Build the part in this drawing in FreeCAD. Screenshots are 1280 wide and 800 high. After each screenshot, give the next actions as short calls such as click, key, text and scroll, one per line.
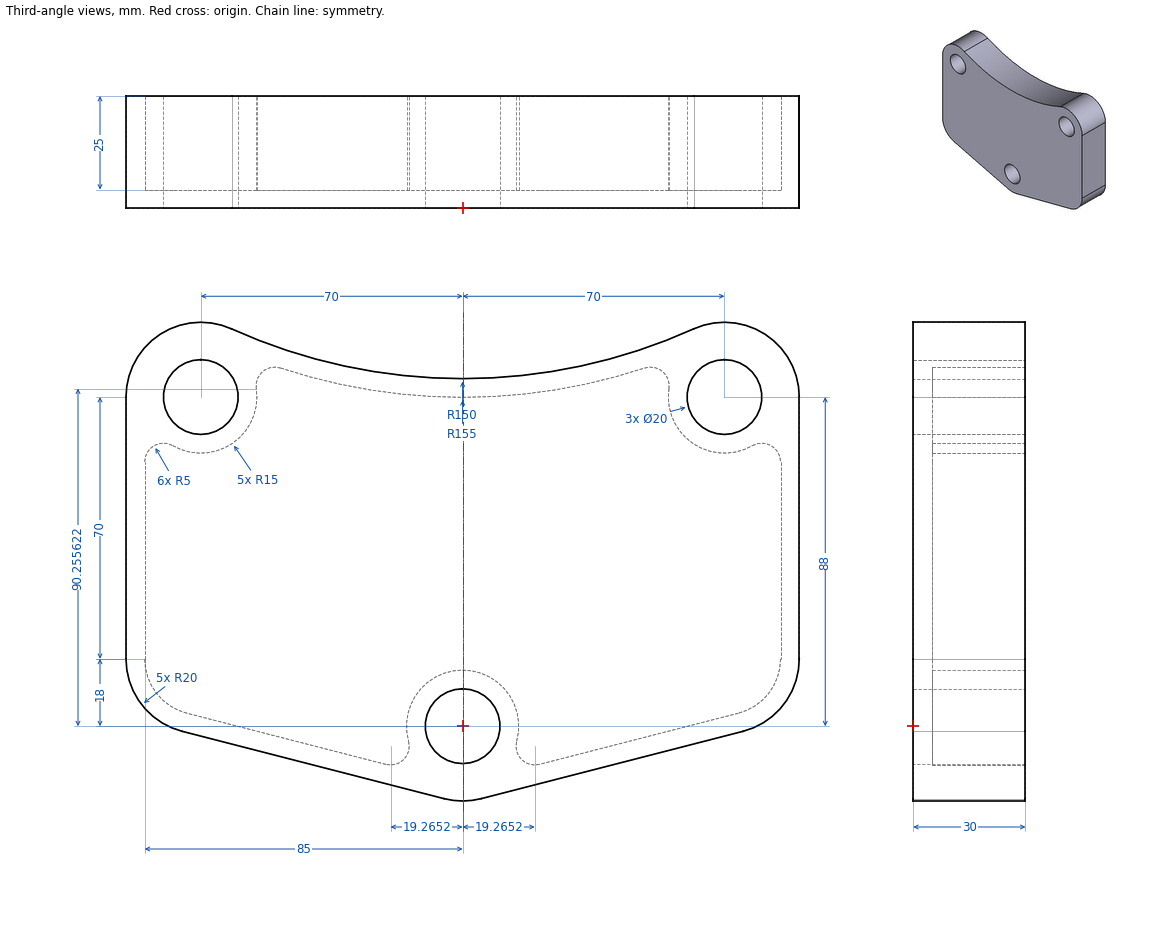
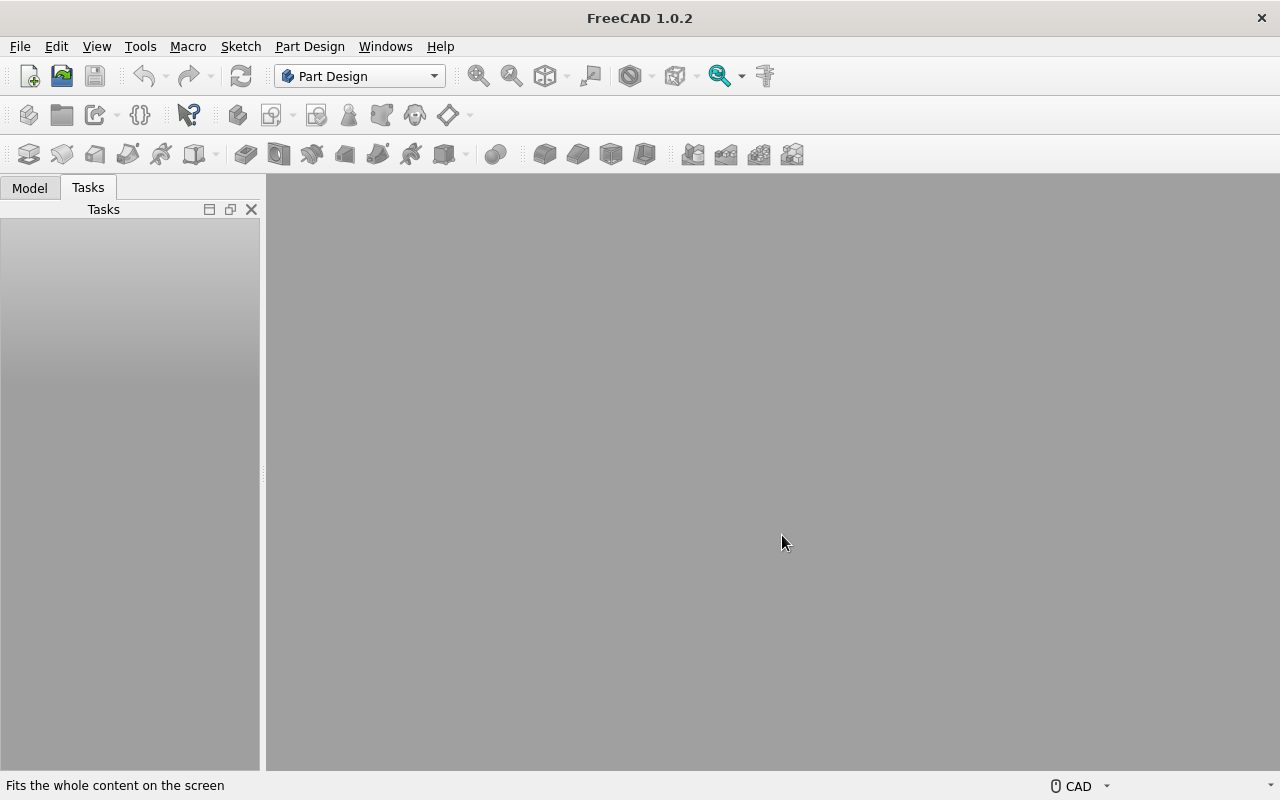
click(29, 76)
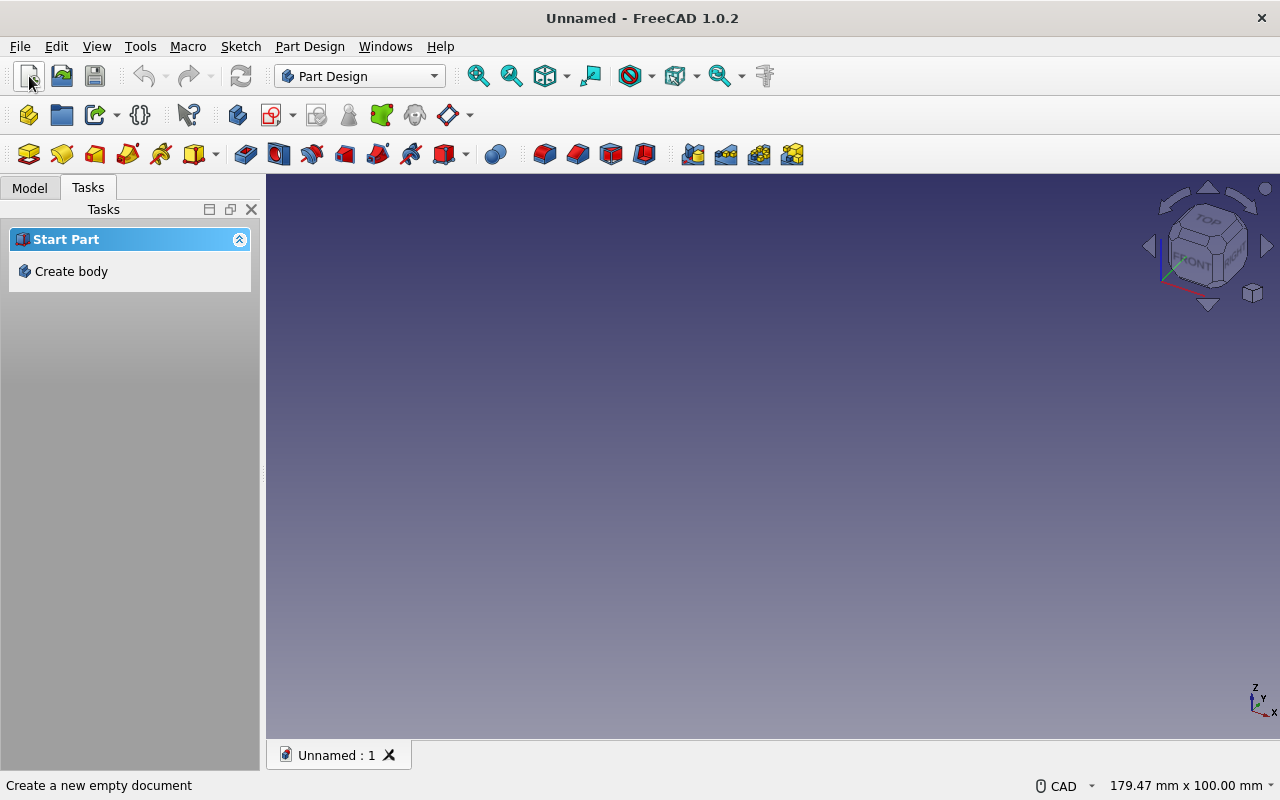
click(270, 116)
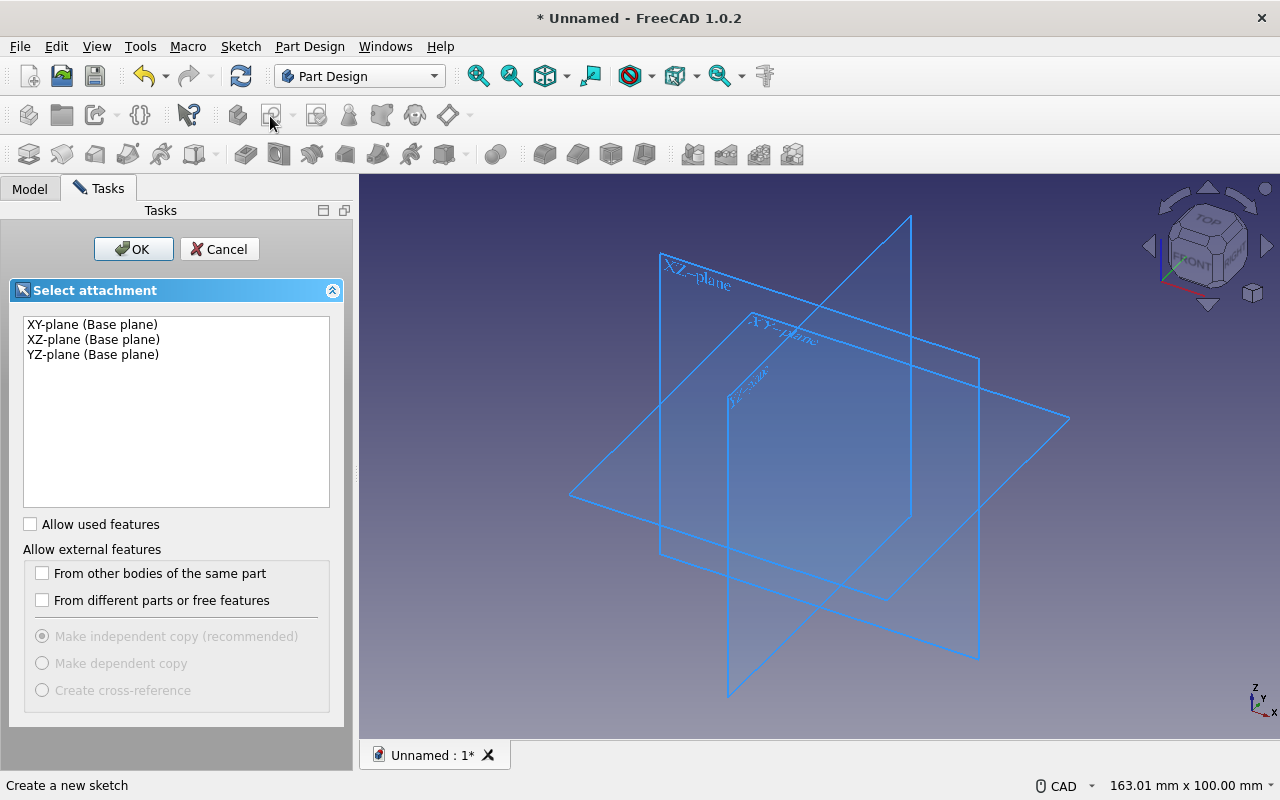
click(84, 340)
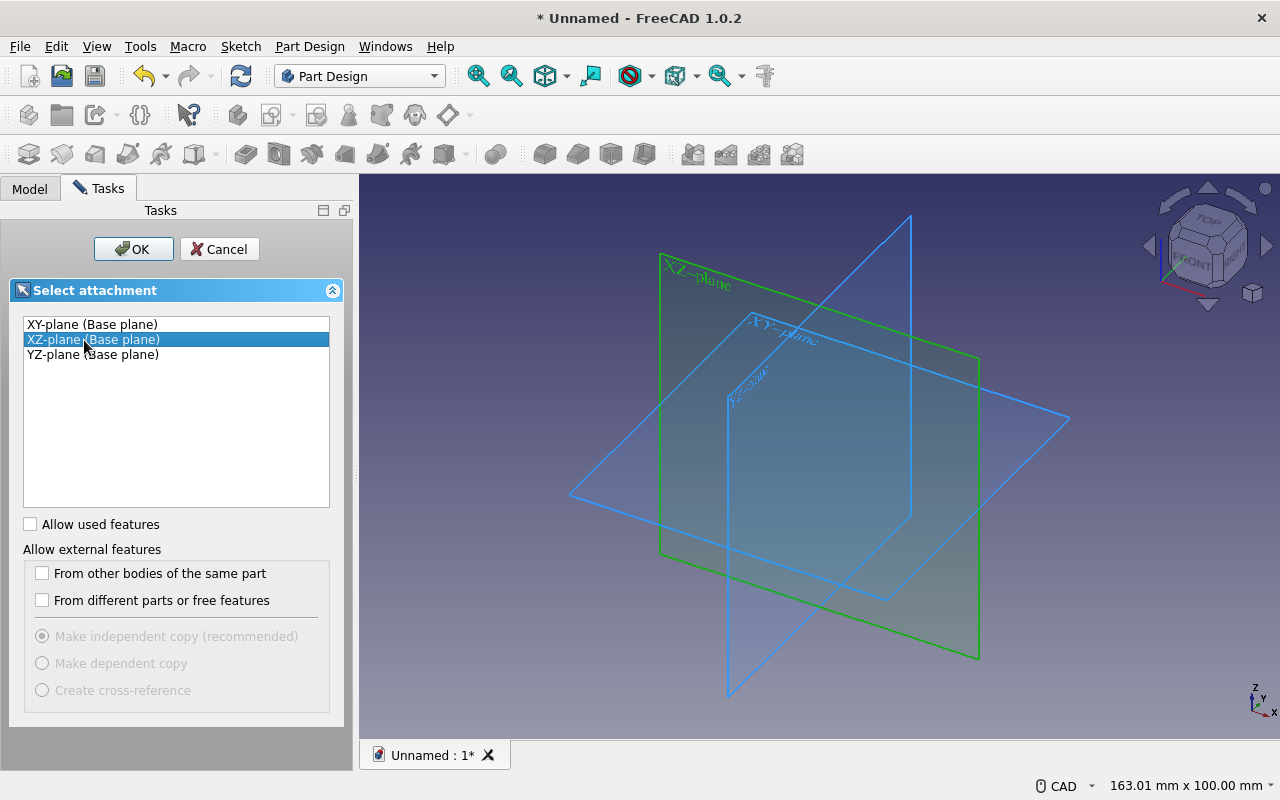
click(134, 249)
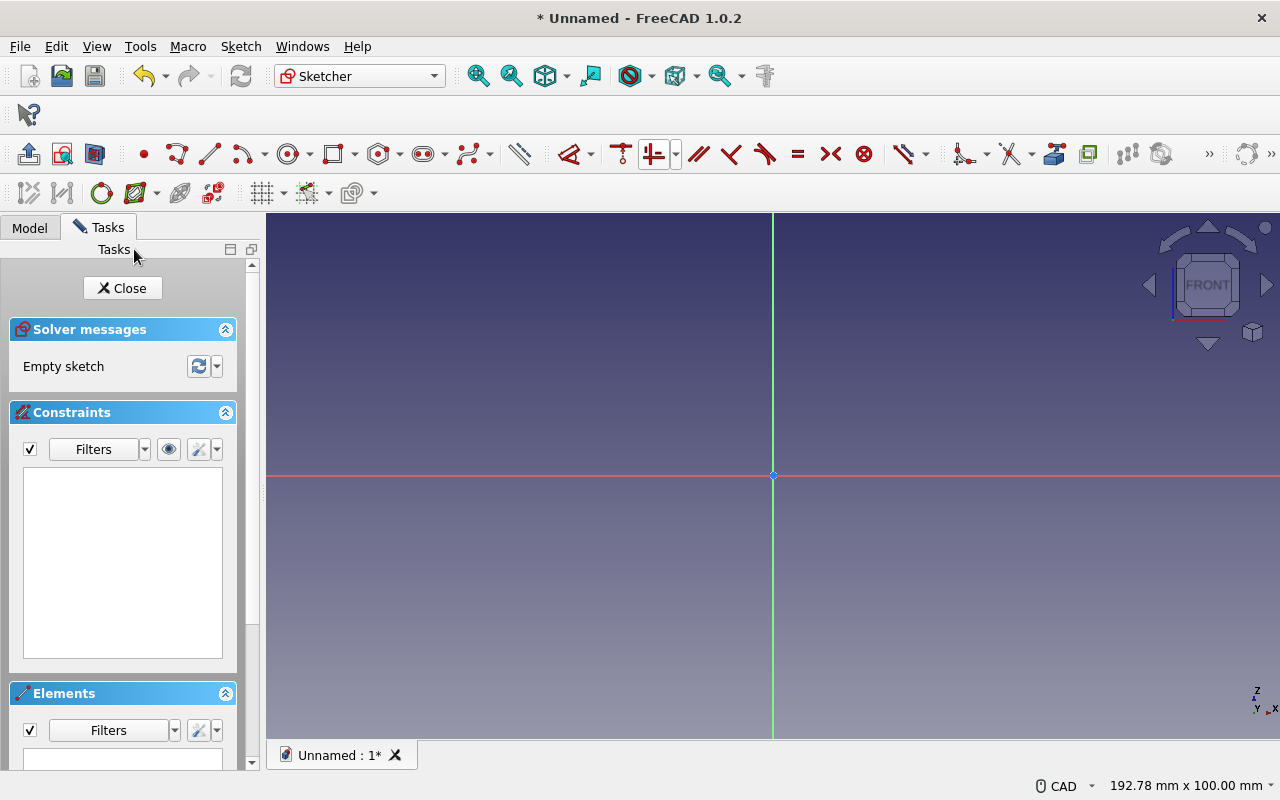
scroll(621, 711, down, 3)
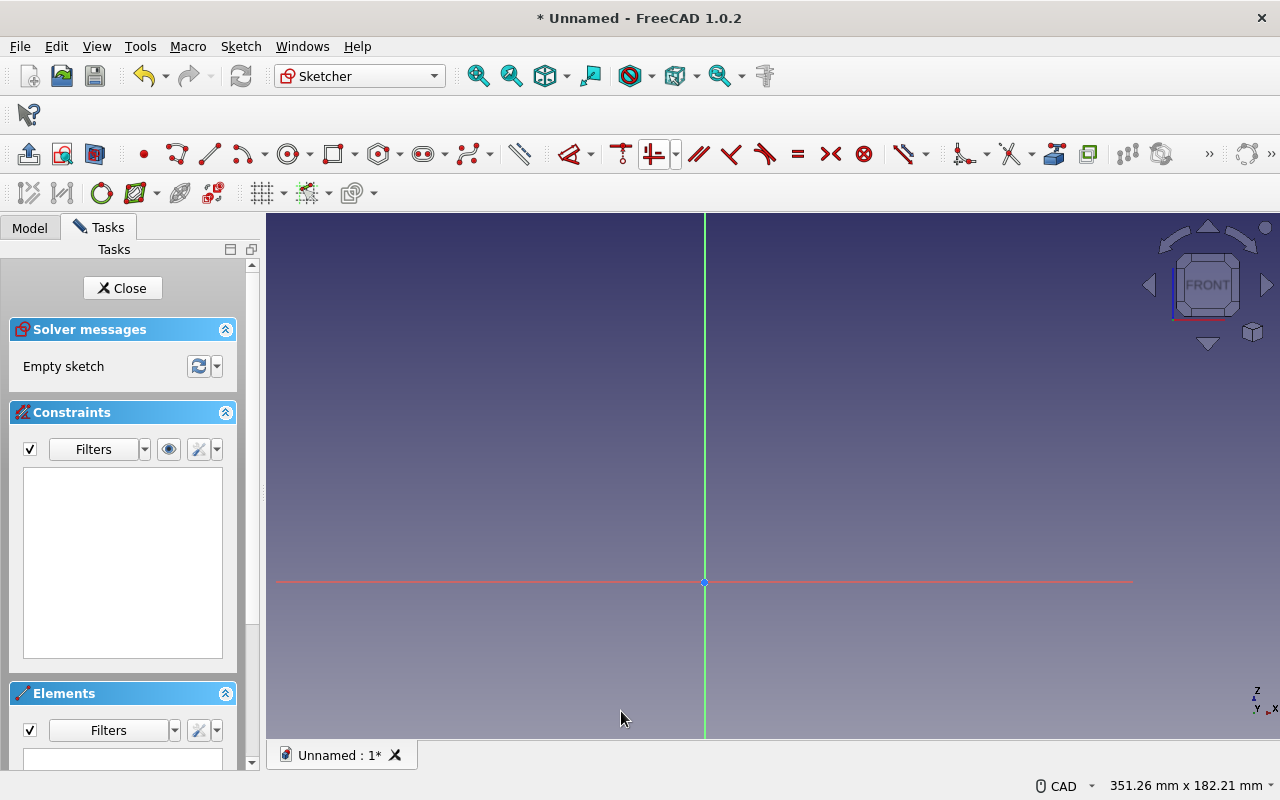
click(210, 154)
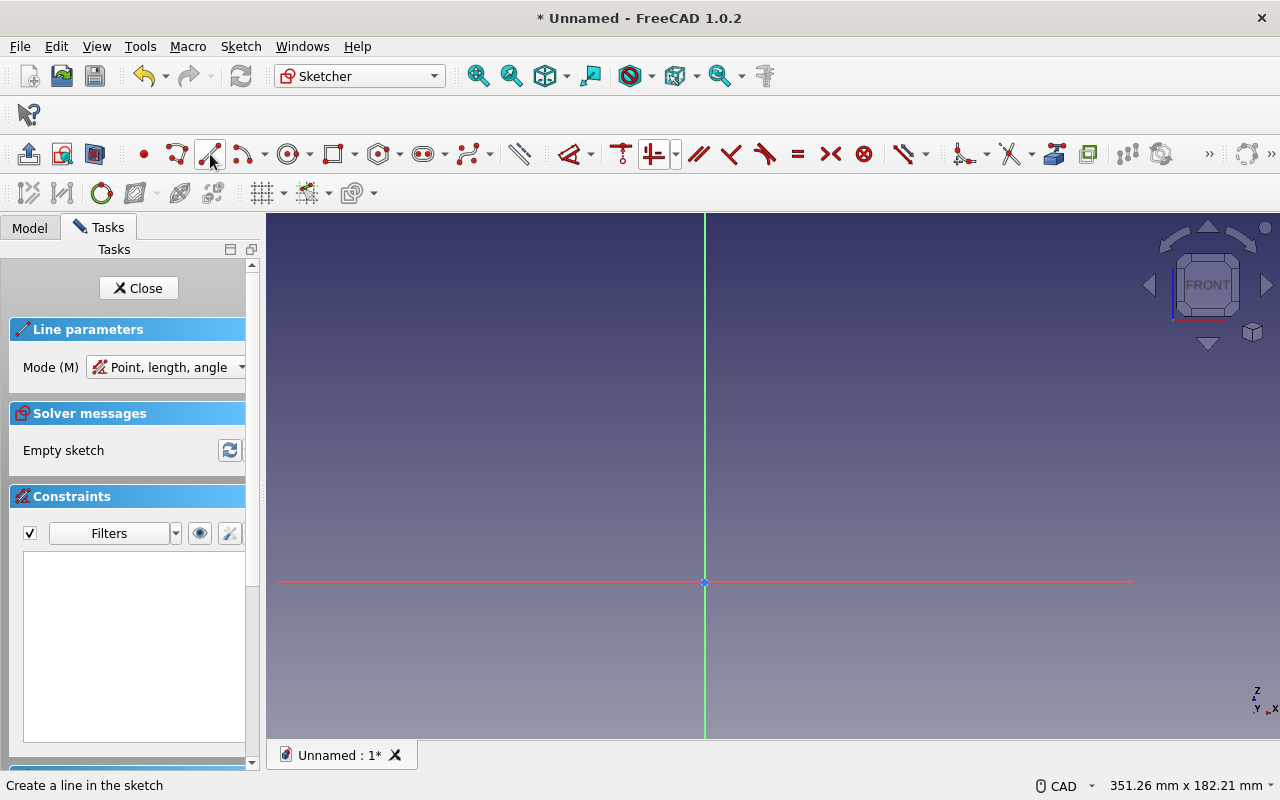
click(690, 638)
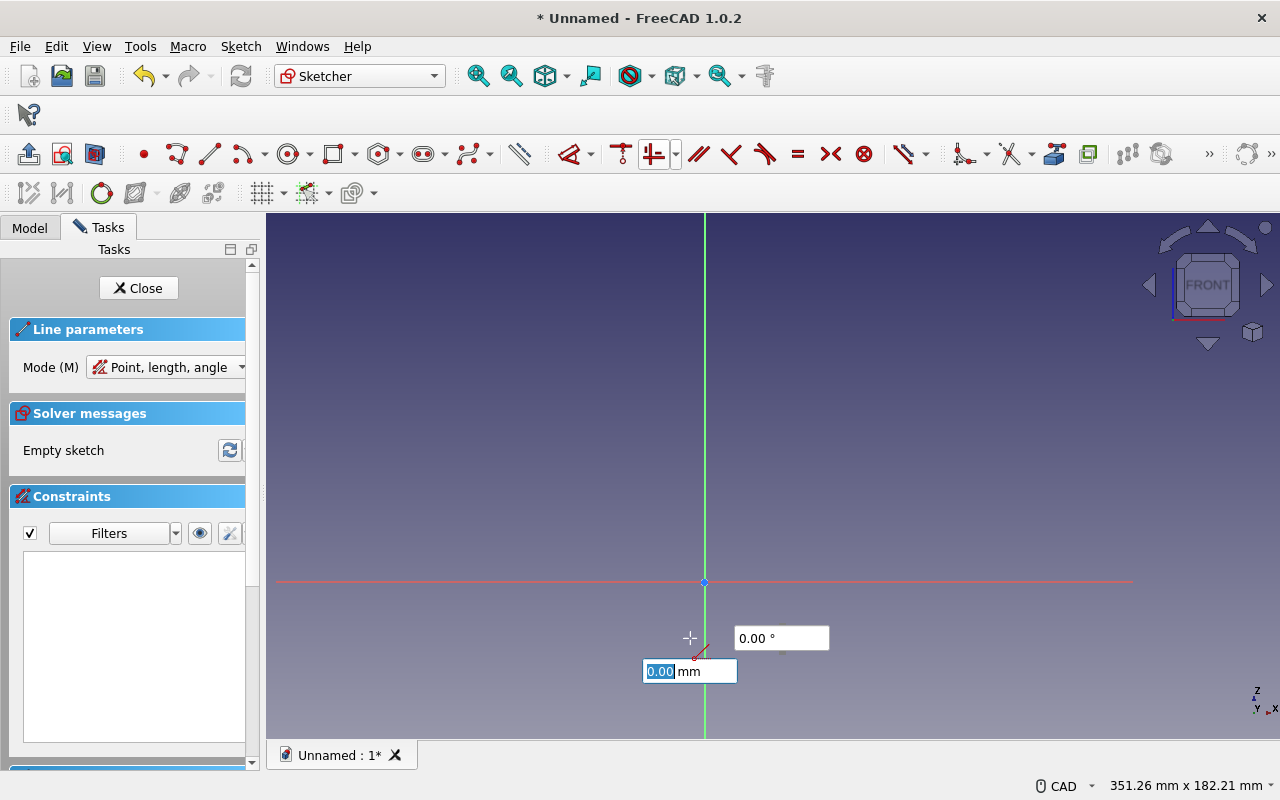
scroll(488, 586, up, 7)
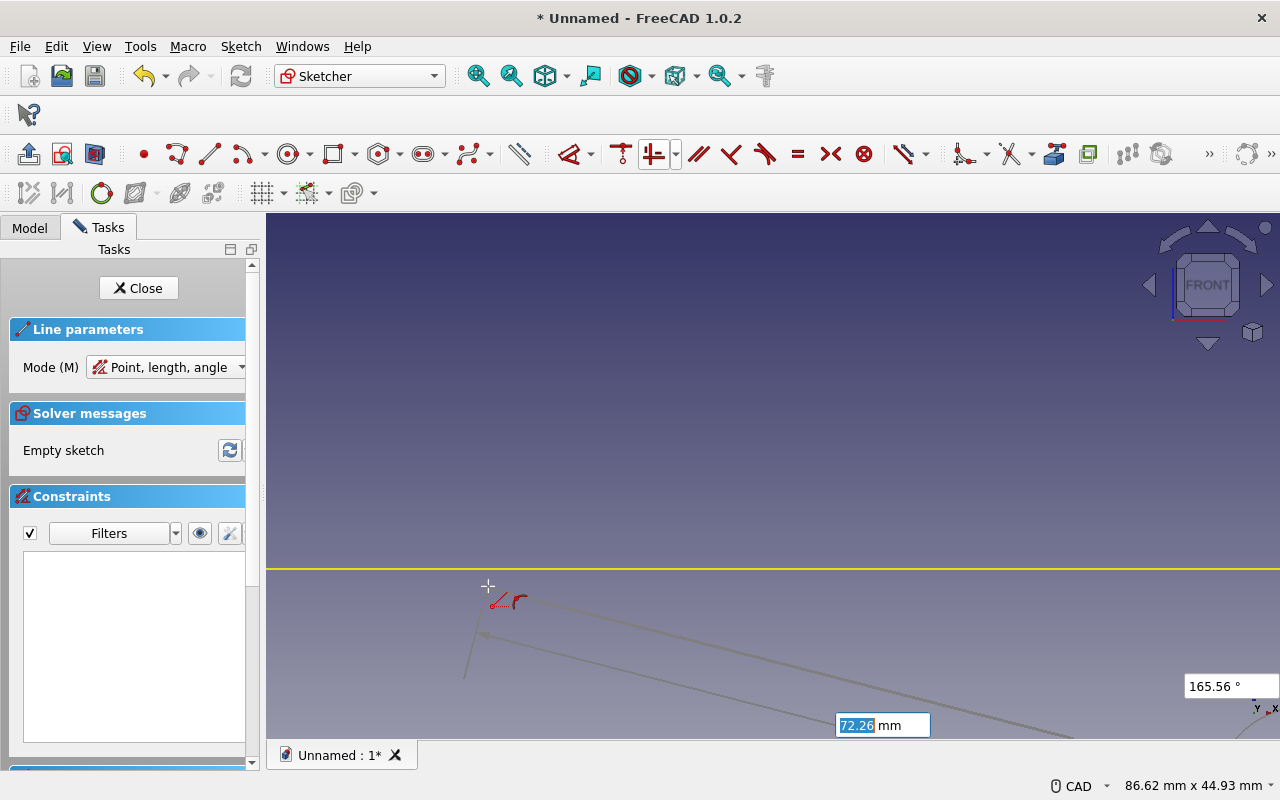
click(488, 585)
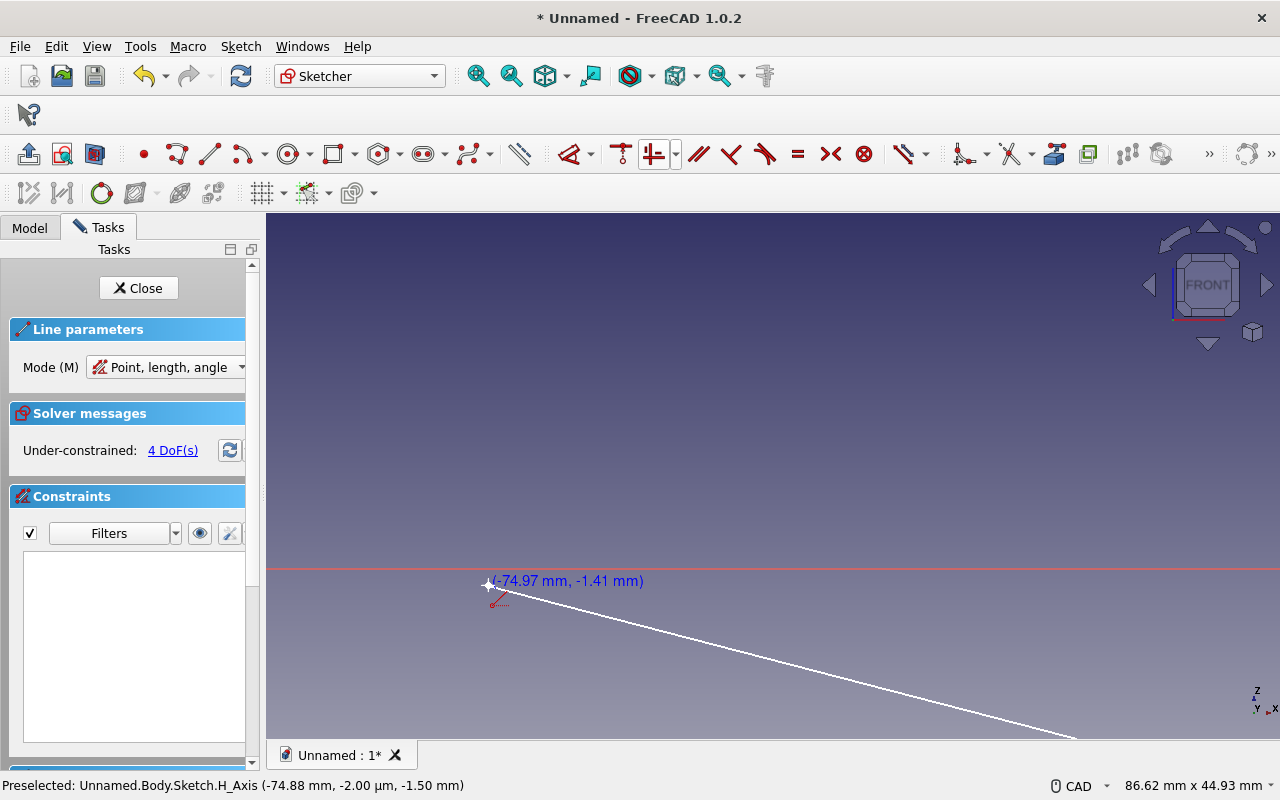
scroll(488, 611, down, 7)